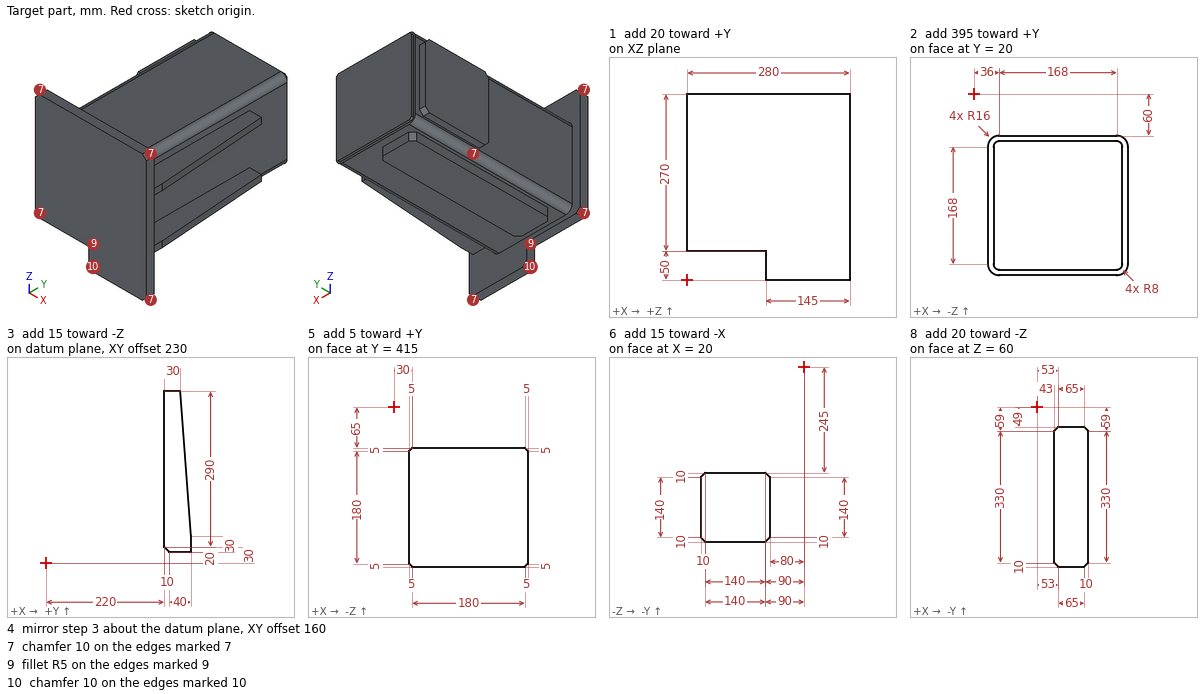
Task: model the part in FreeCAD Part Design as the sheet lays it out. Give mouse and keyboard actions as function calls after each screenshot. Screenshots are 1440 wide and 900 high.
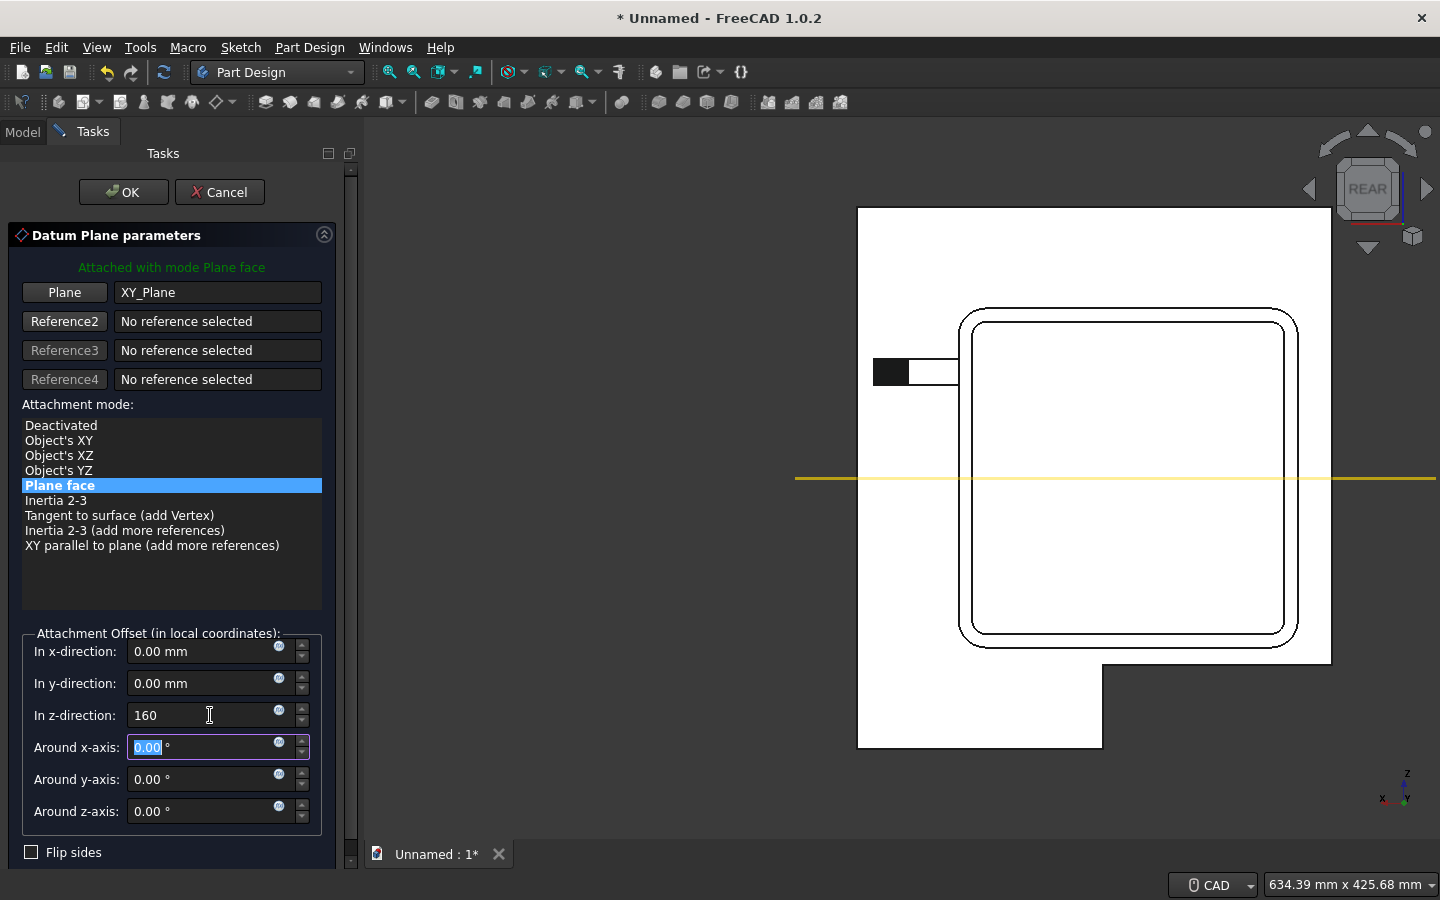
click(124, 192)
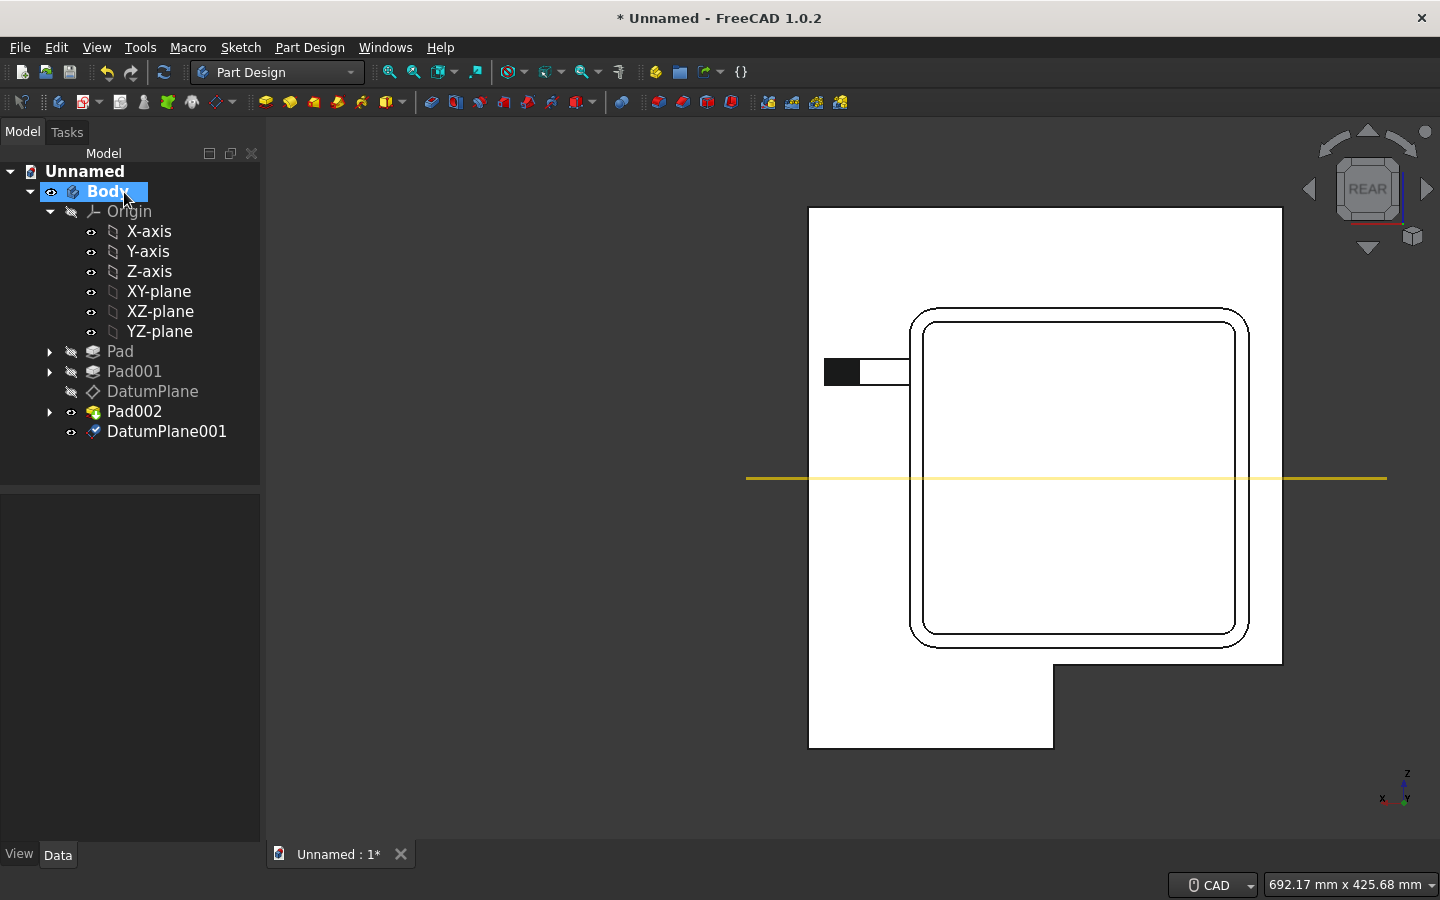
click(116, 412)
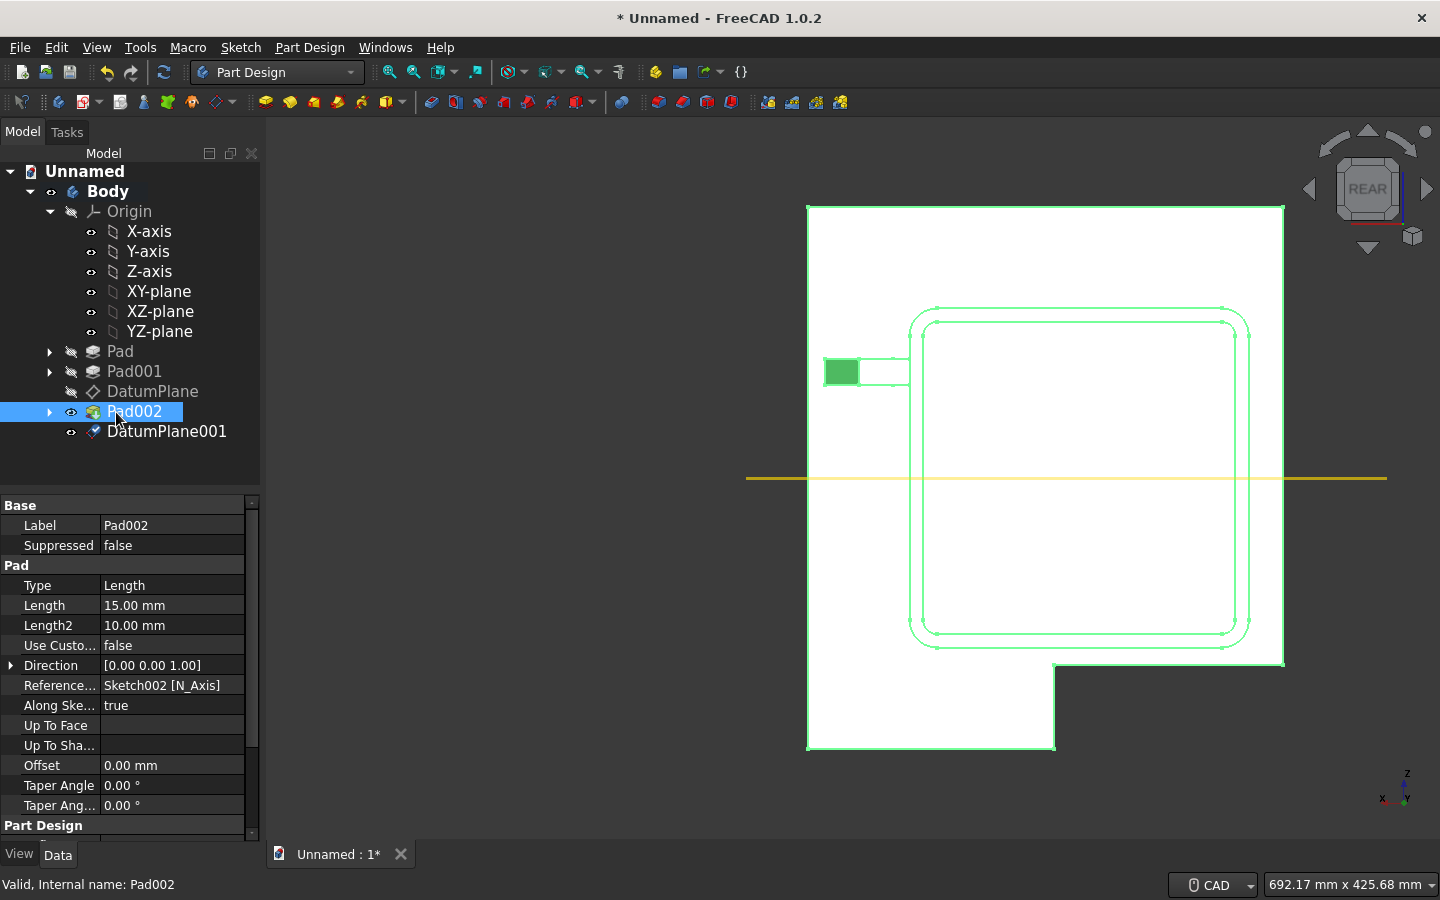
click(768, 102)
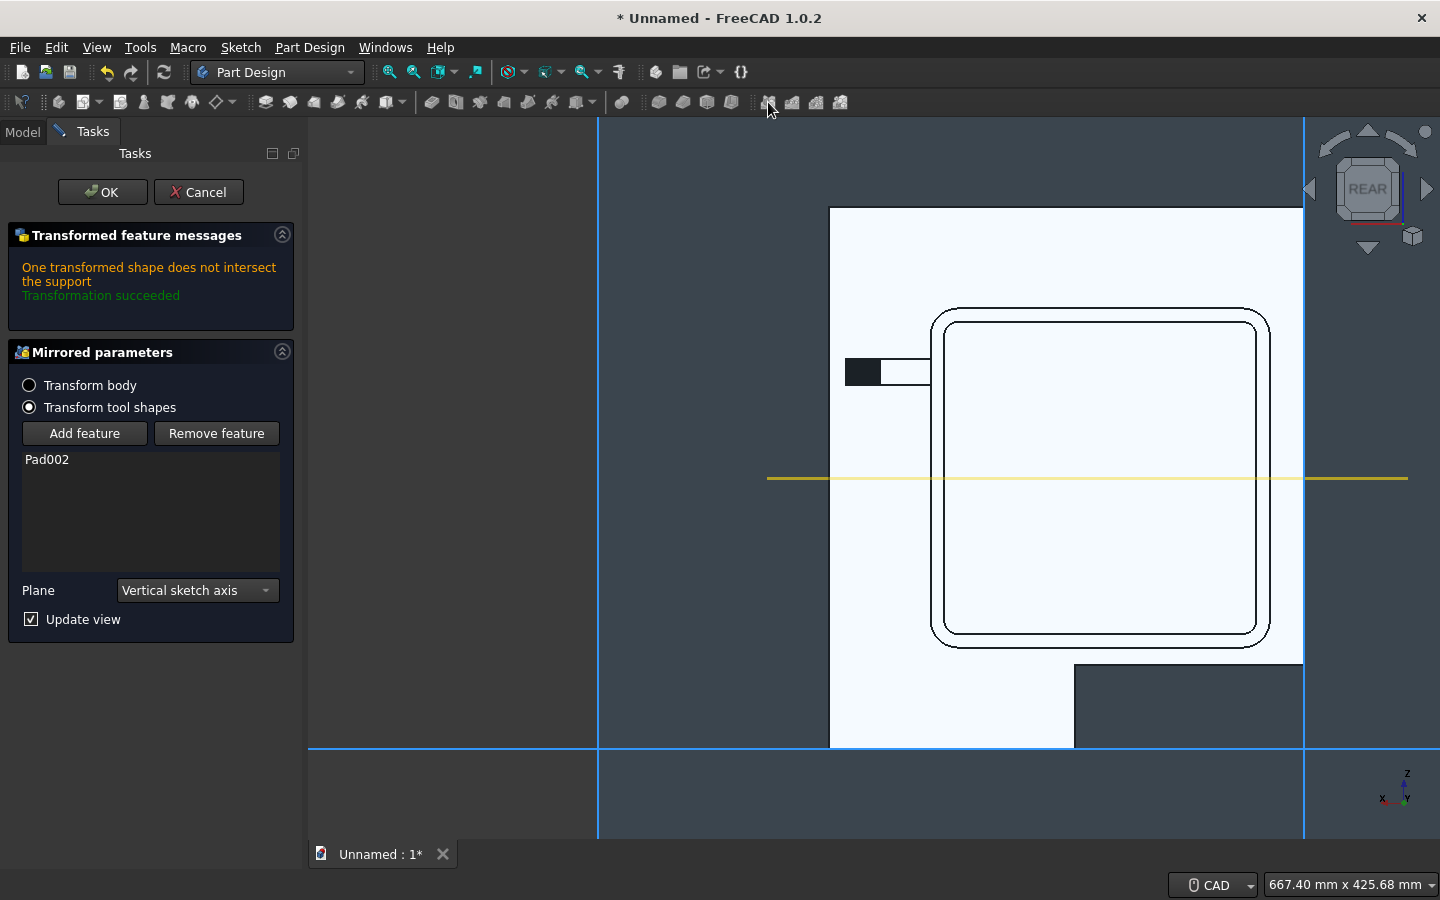
click(198, 590)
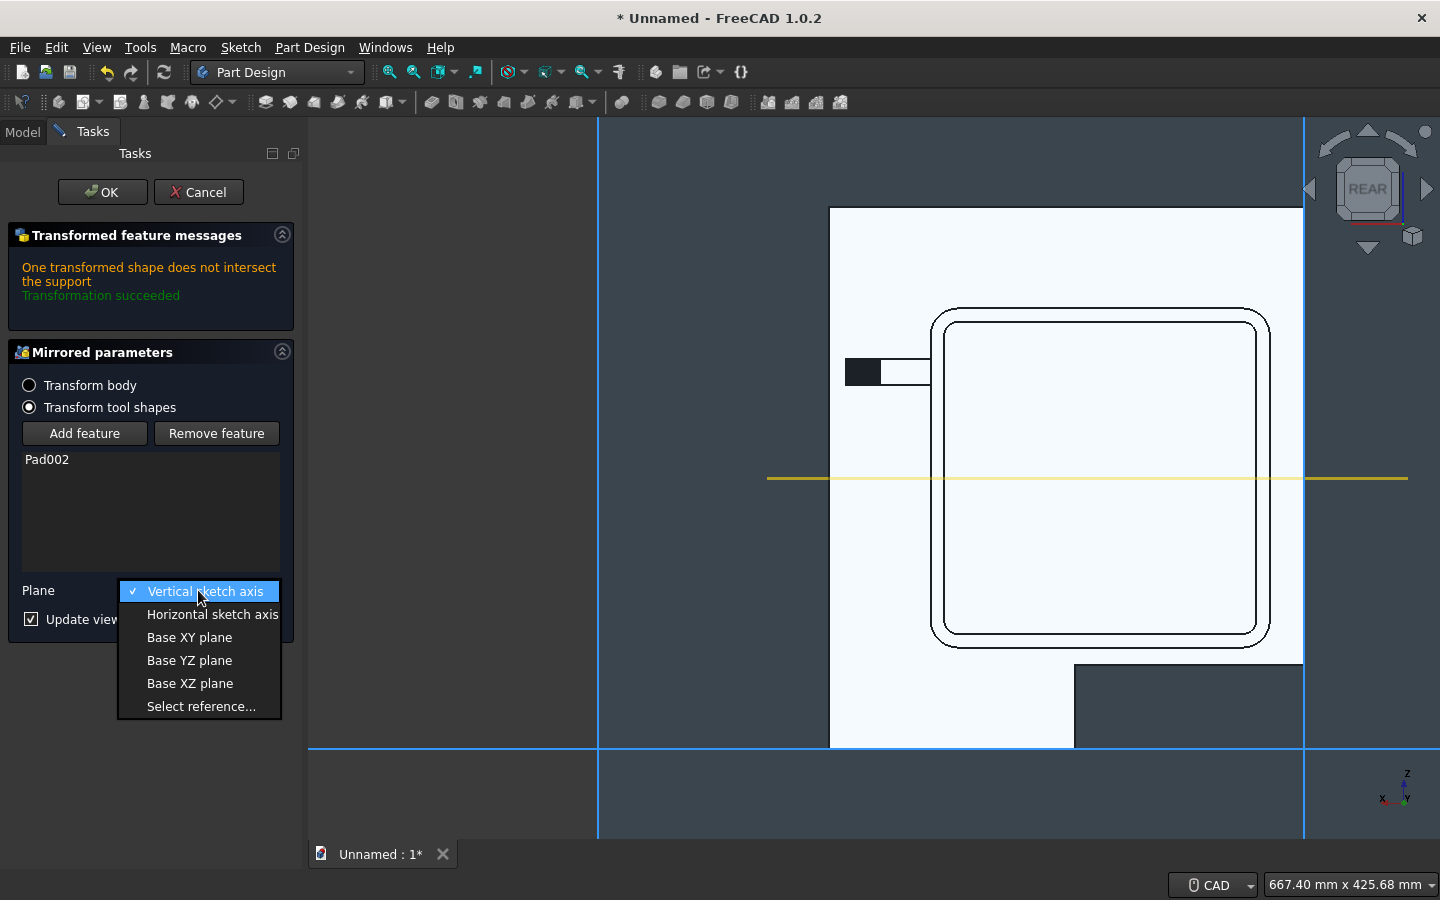
click(198, 706)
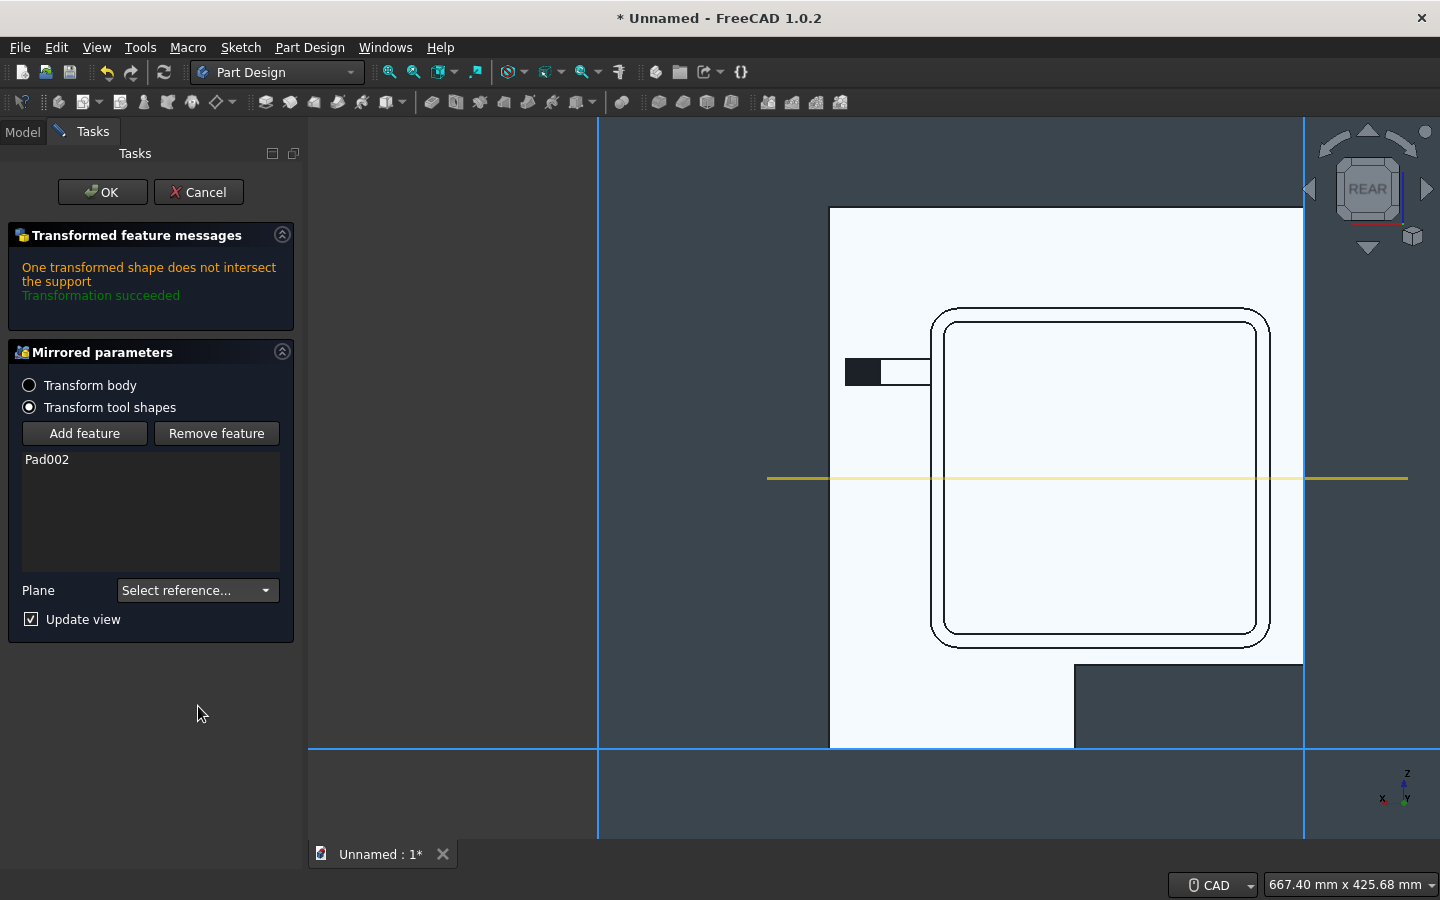
click(23, 131)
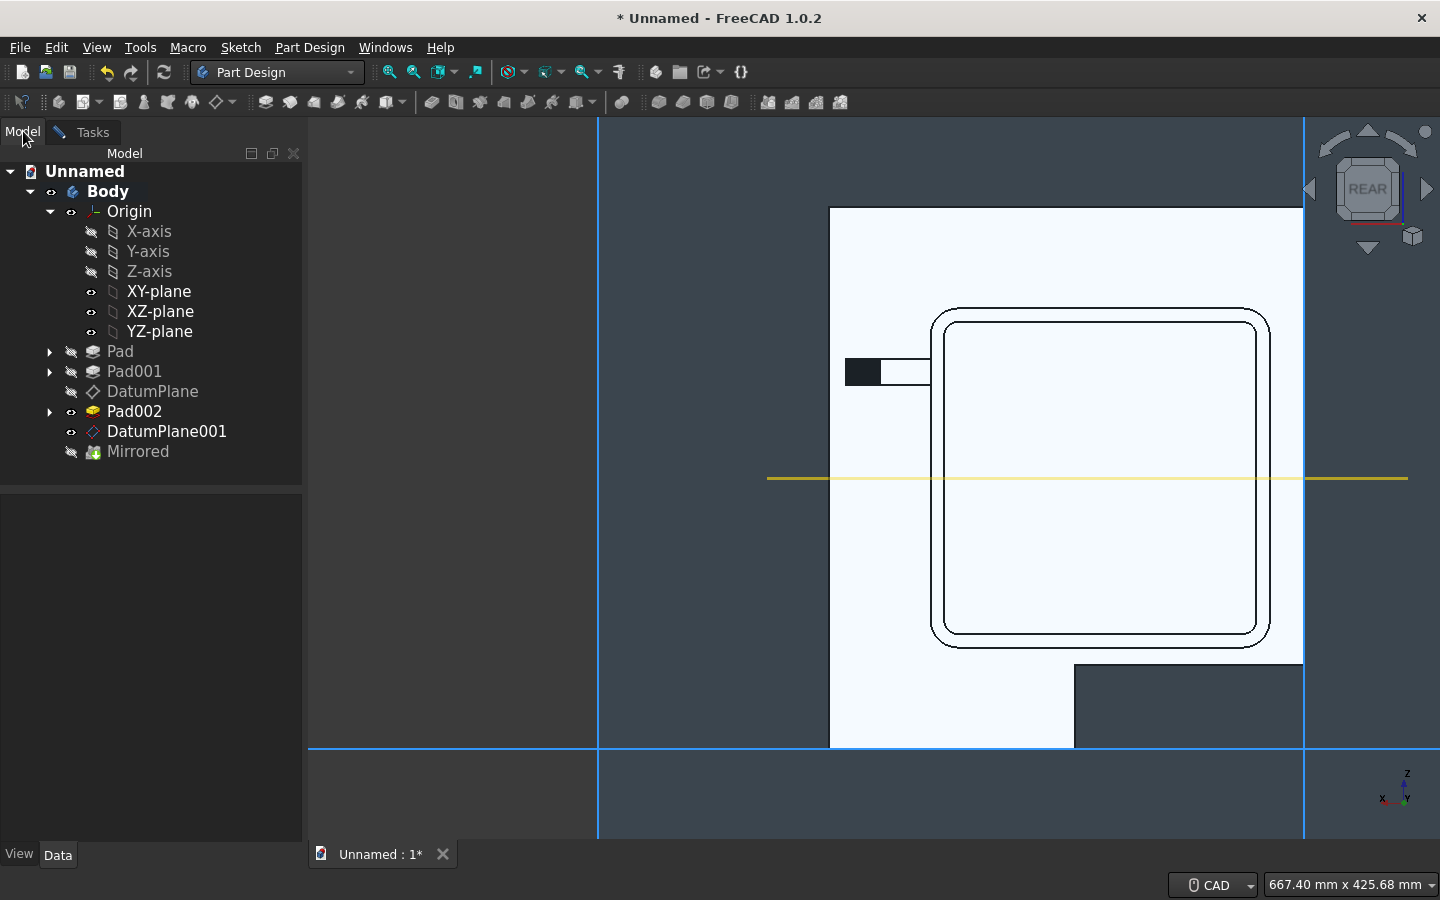
click(116, 432)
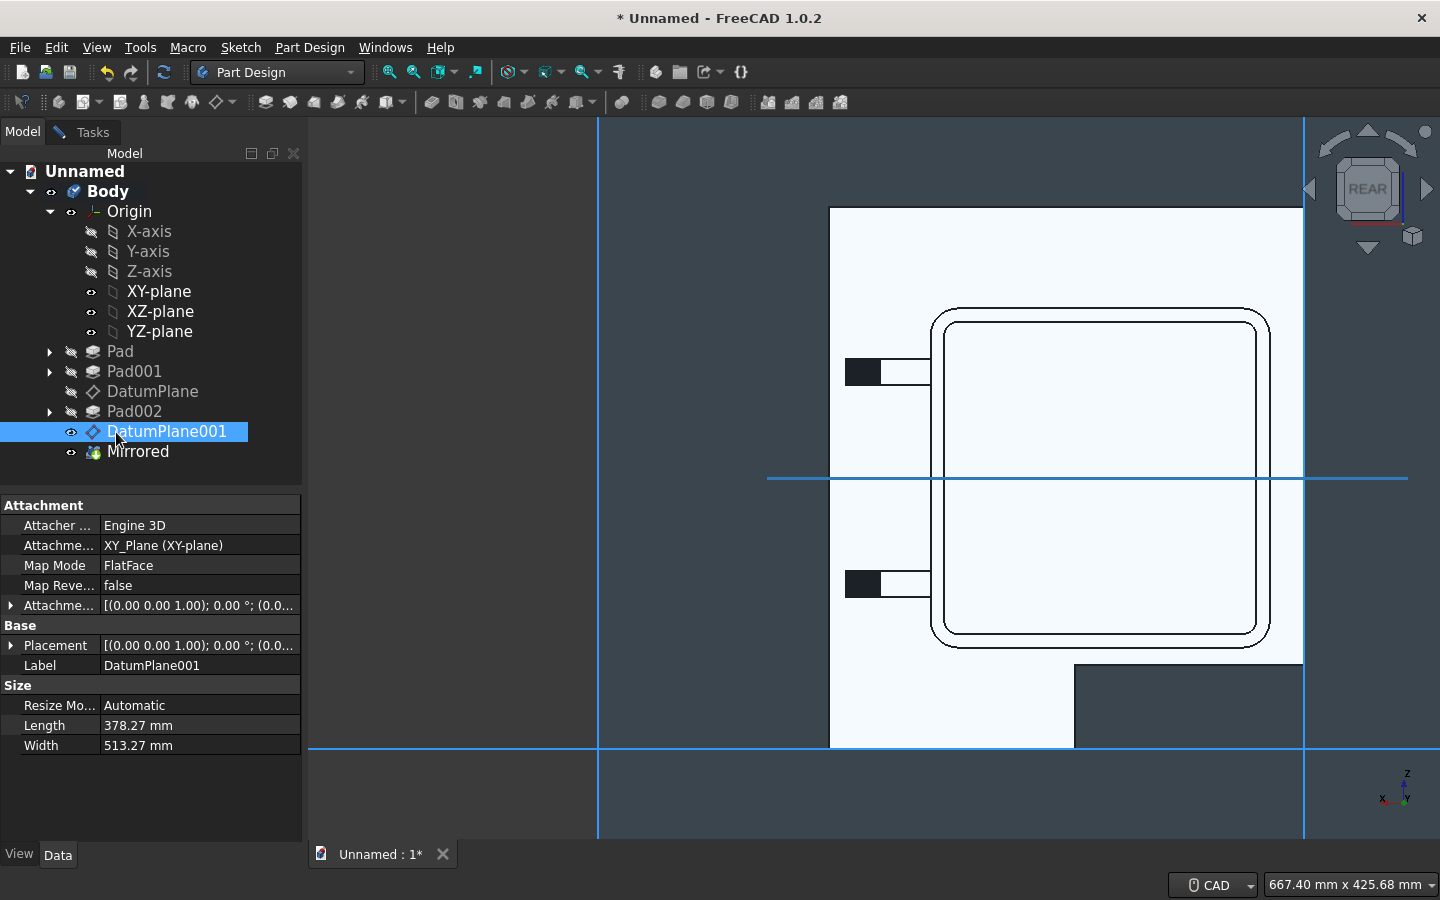
click(84, 131)